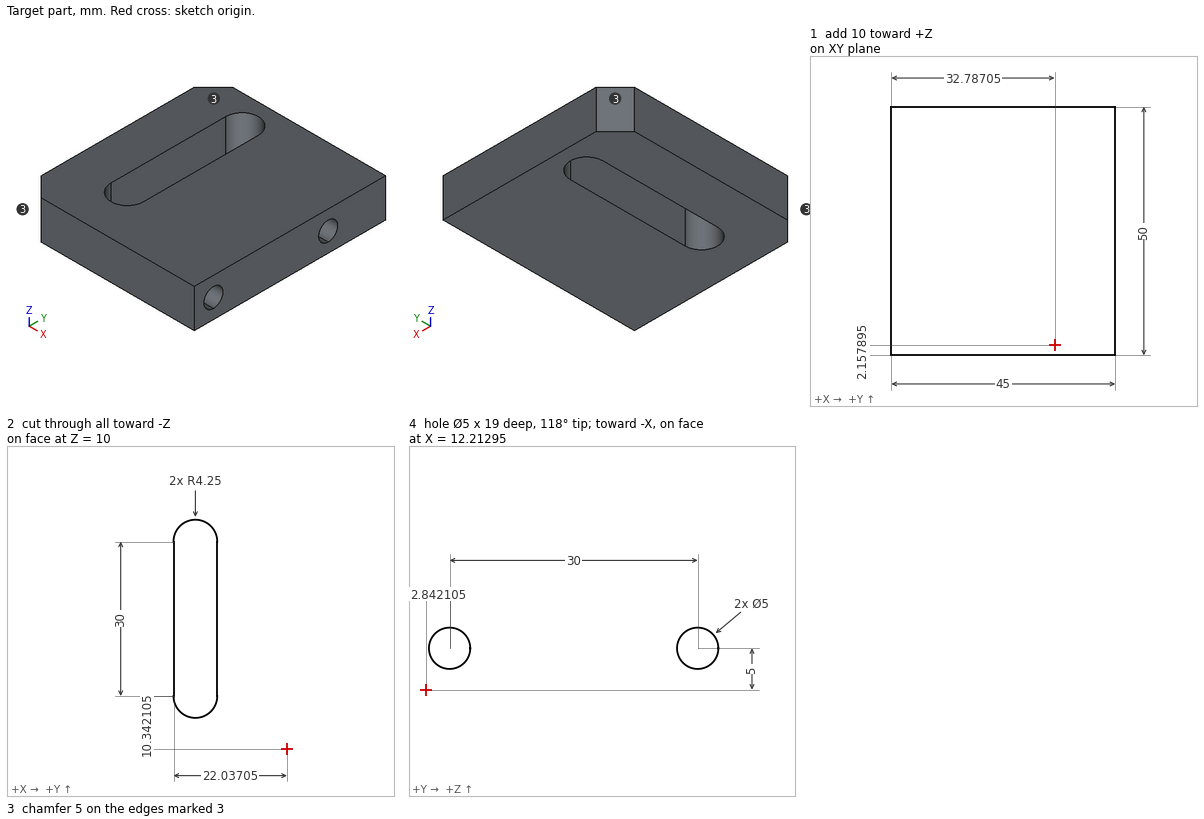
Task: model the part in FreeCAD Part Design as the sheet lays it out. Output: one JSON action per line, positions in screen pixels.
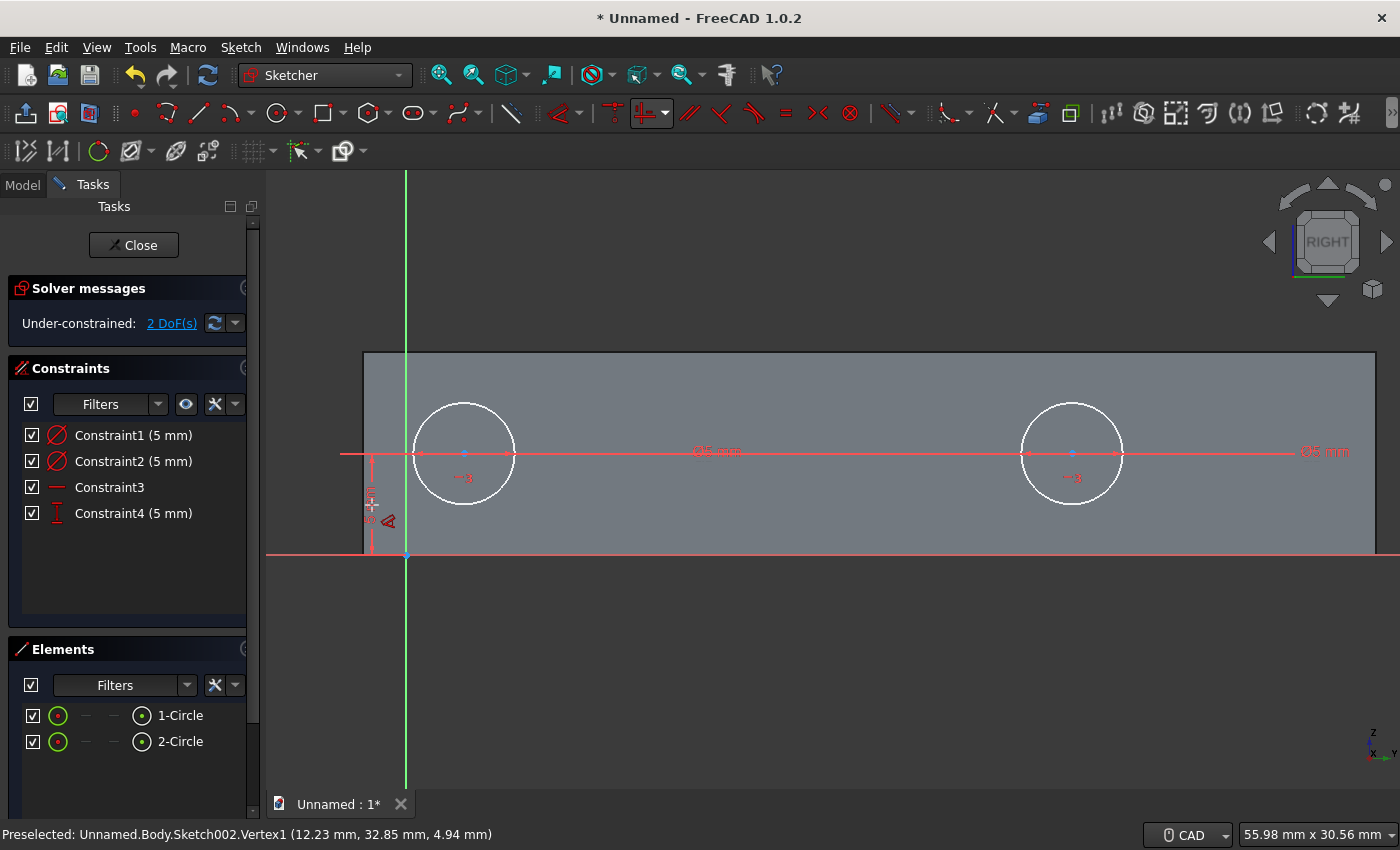
{"action": "left_click", "coordinate": [1072, 454]}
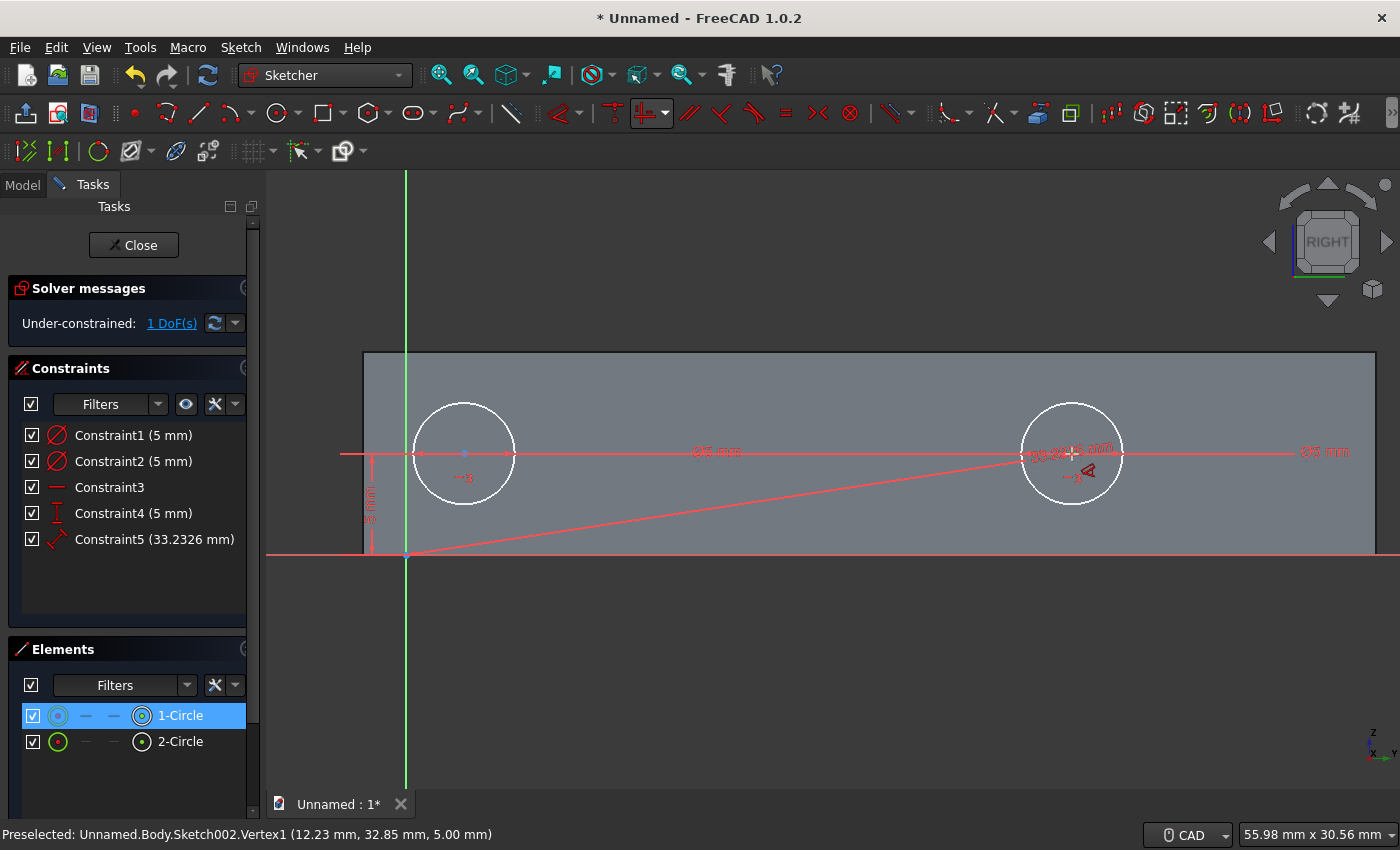
{"action": "left_click", "coordinate": [464, 454]}
{"action": "left_click", "coordinate": [768, 420]}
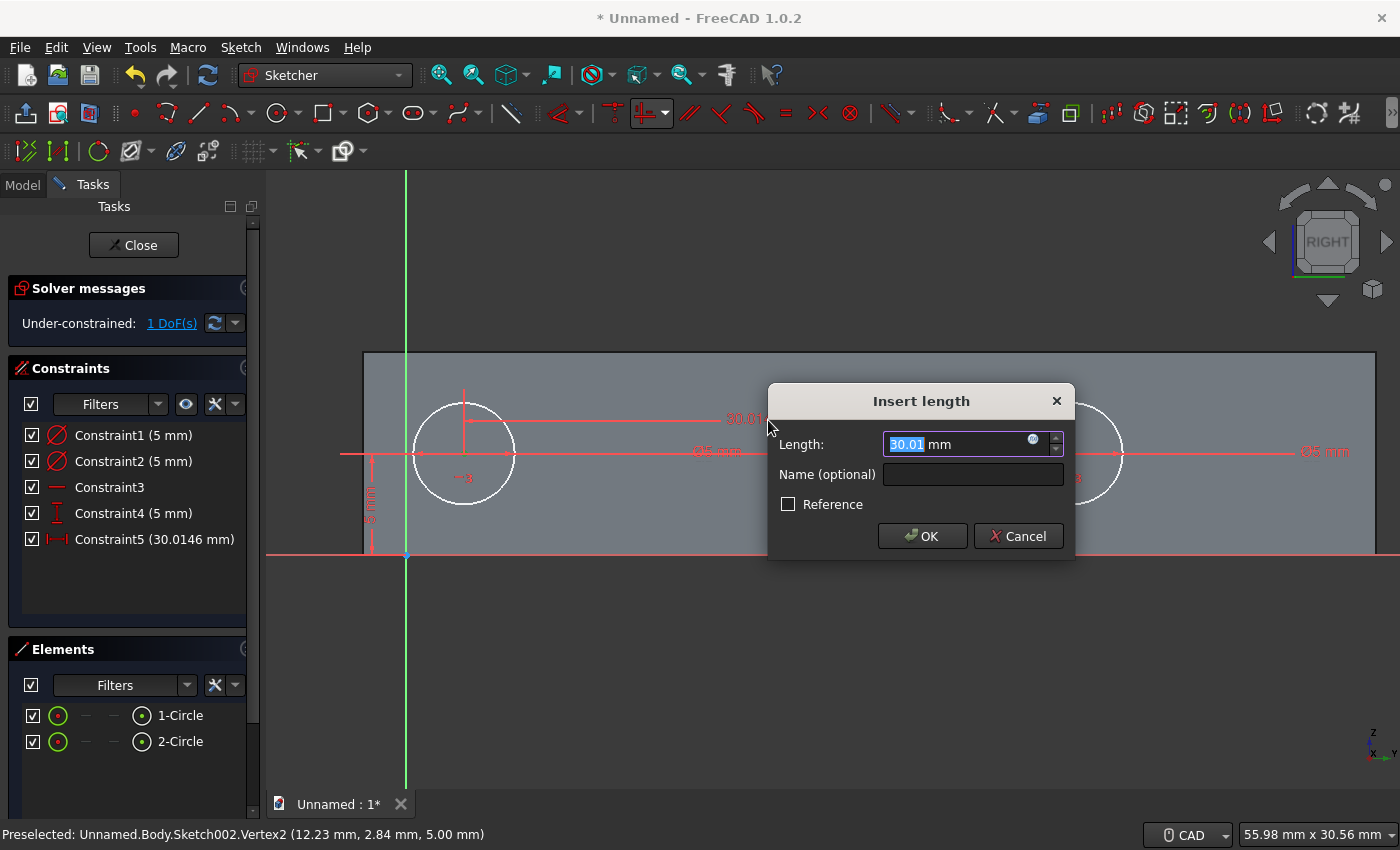
{"action": "type", "text": "30"}
{"action": "key", "text": "Return"}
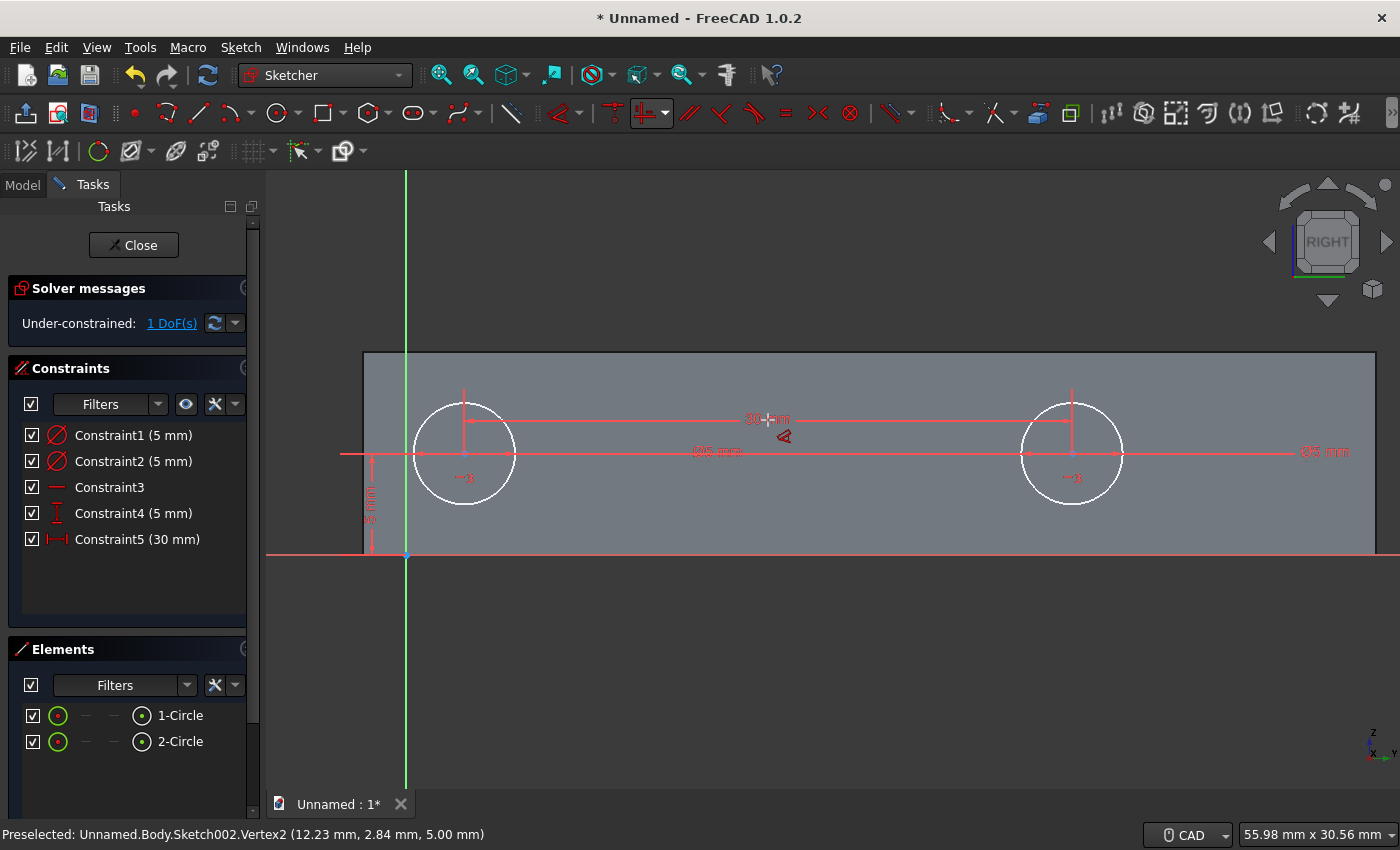
{"action": "left_click", "coordinate": [464, 454]}
{"action": "left_click", "coordinate": [435, 589]}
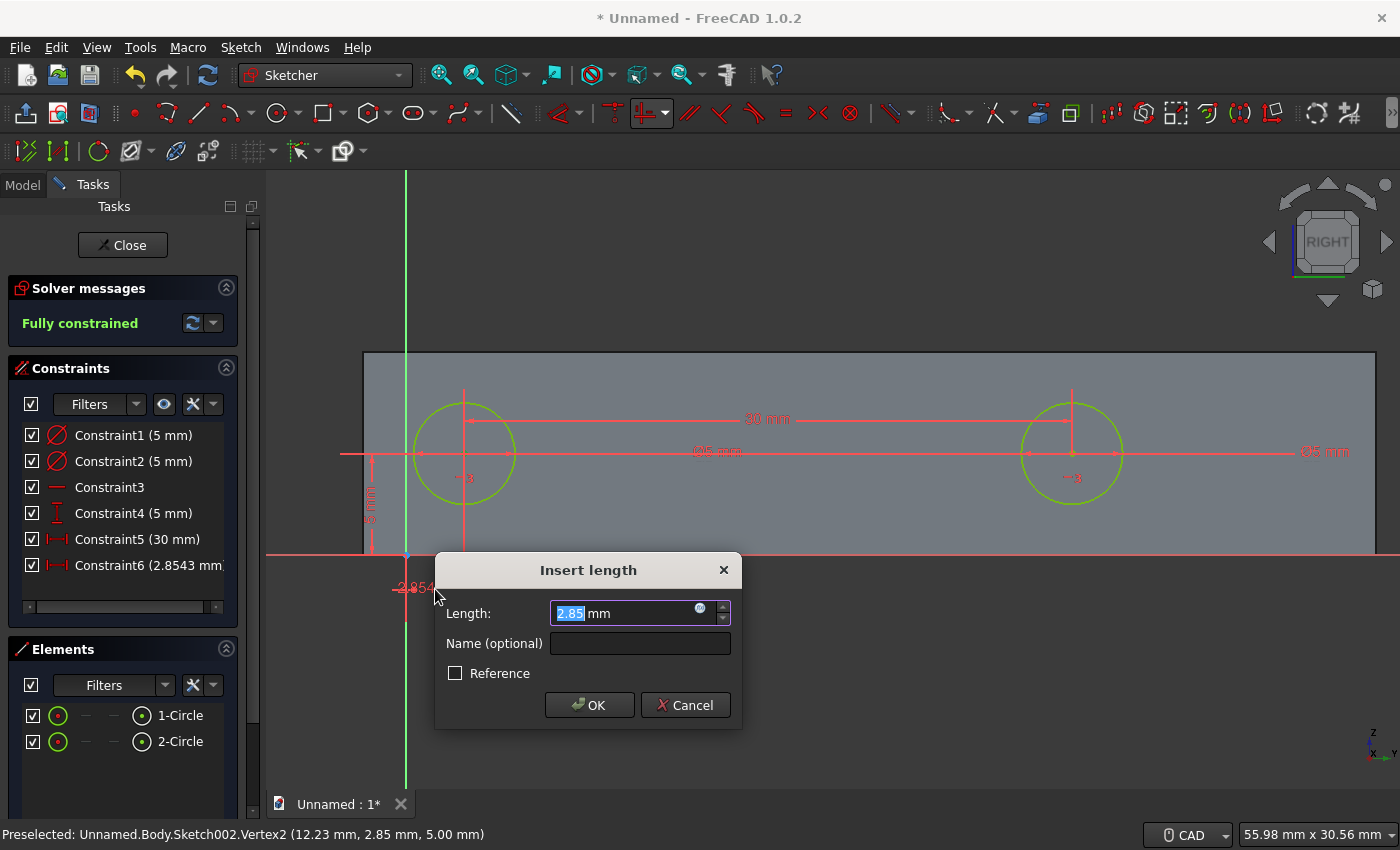
{"action": "type", "text": "2.842105"}
{"action": "key", "text": "Return"}
{"action": "key", "text": "Escape"}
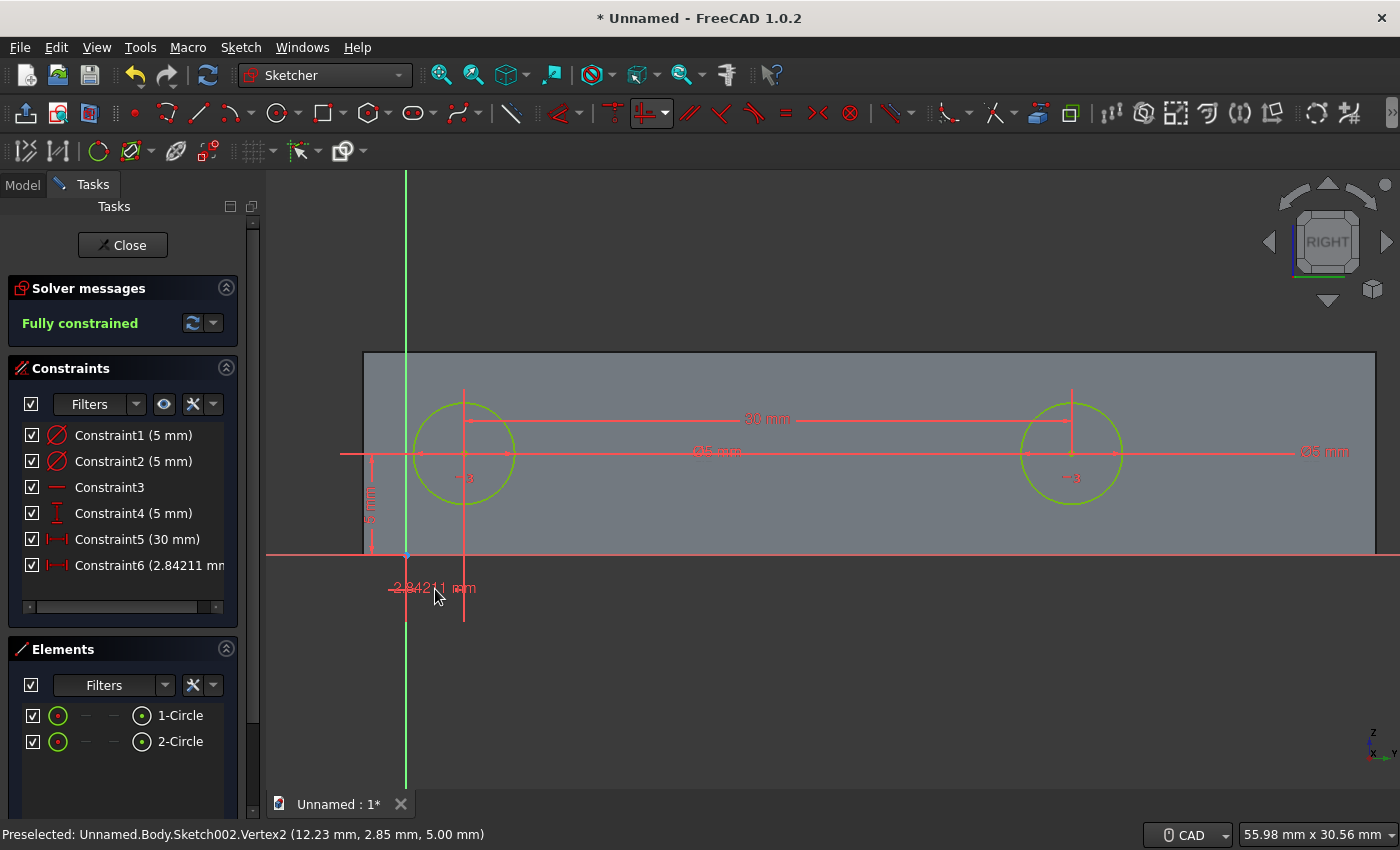
{"action": "left_click", "coordinate": [123, 245]}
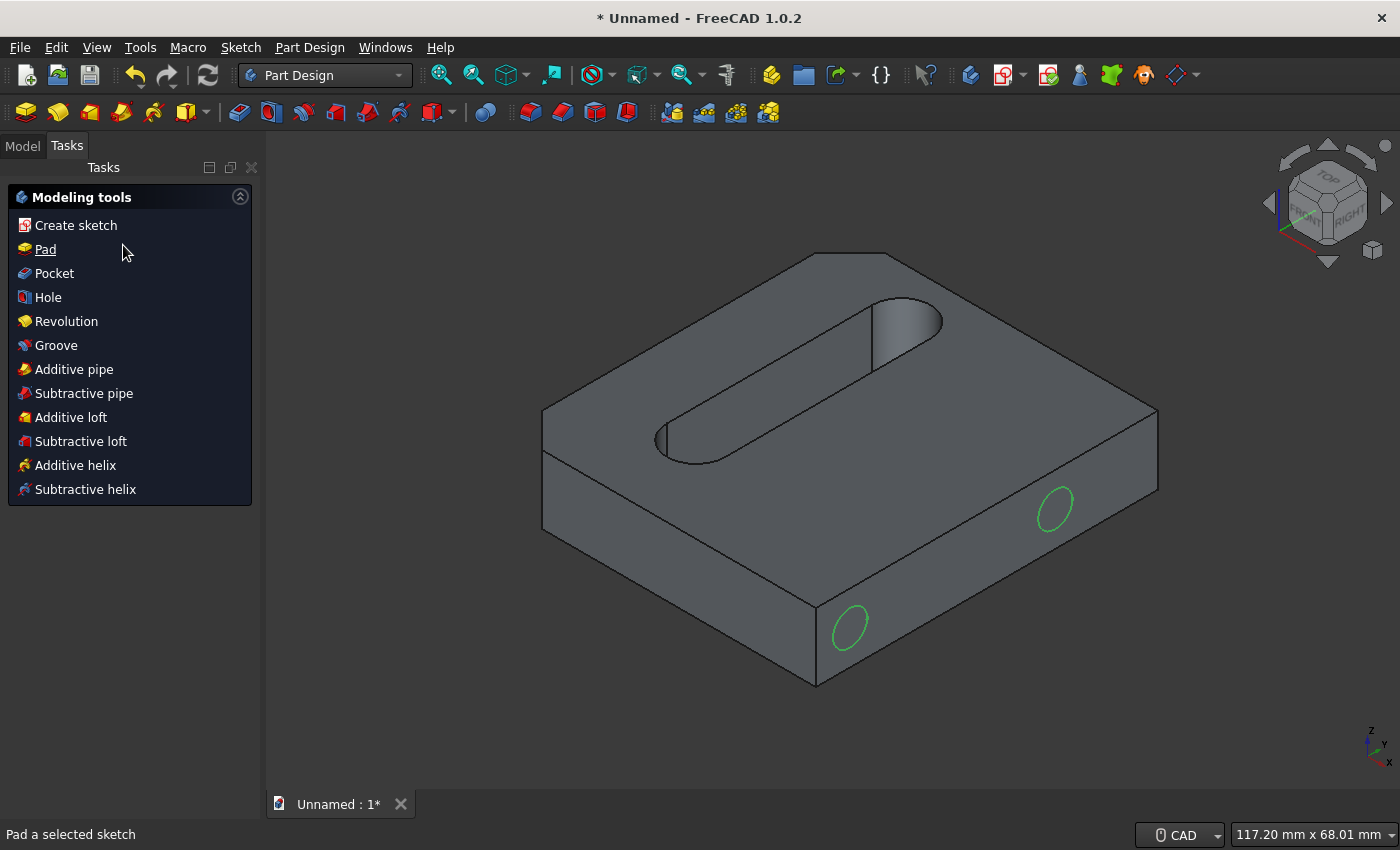
{"action": "left_click", "coordinate": [272, 112]}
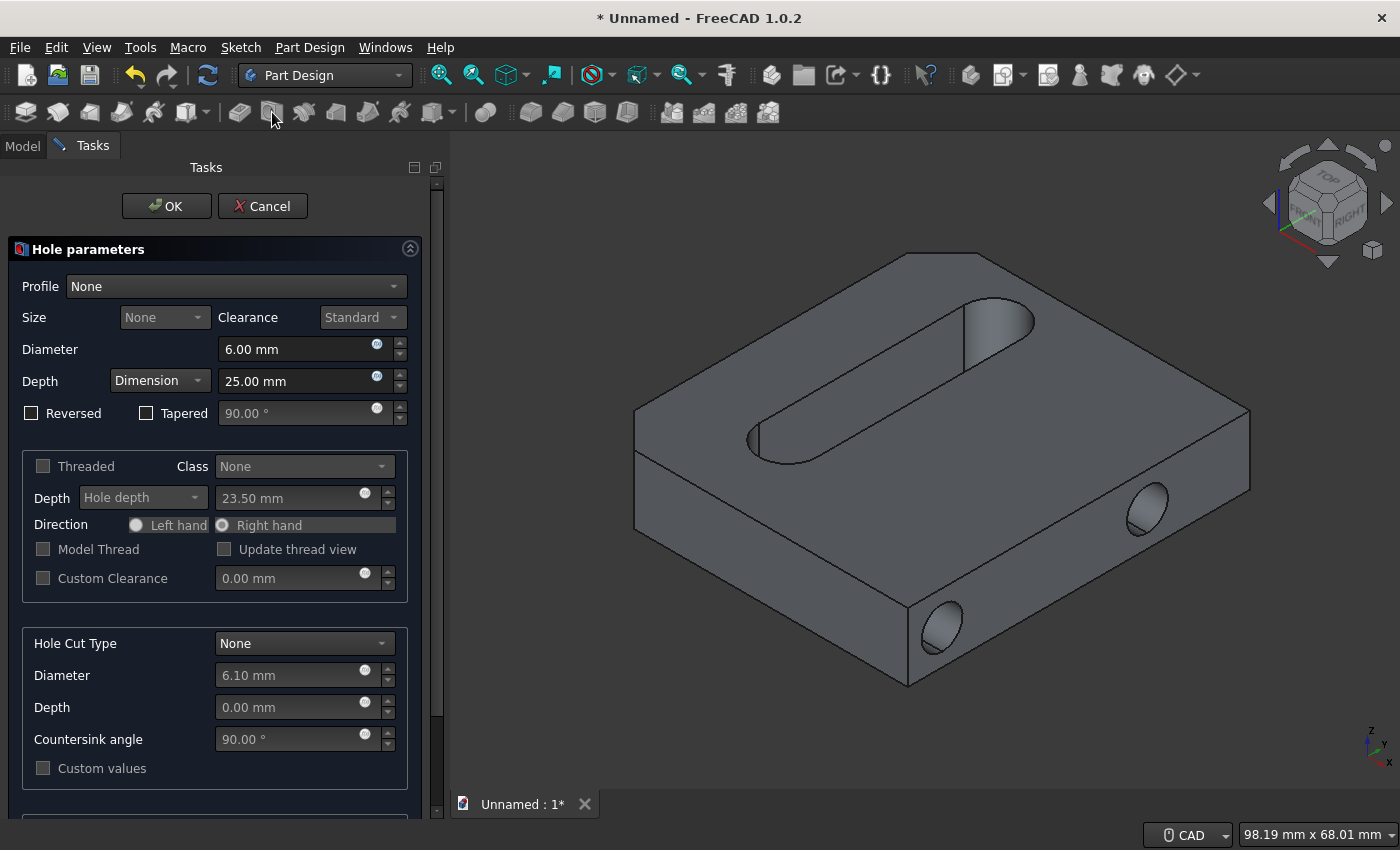
{"action": "triple_click", "coordinate": [305, 349]}